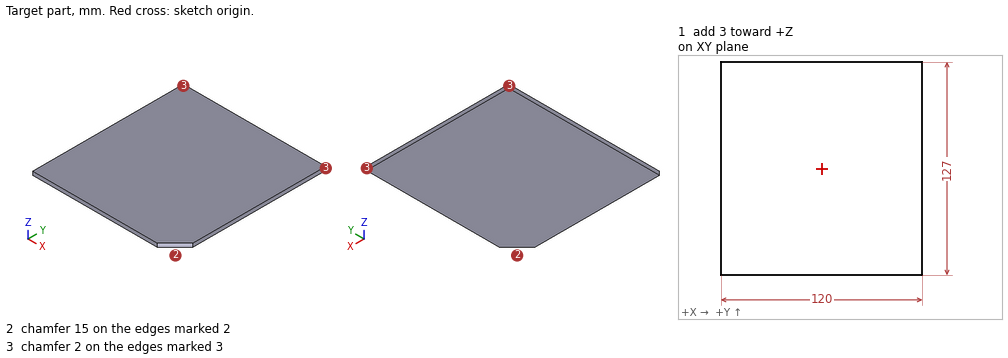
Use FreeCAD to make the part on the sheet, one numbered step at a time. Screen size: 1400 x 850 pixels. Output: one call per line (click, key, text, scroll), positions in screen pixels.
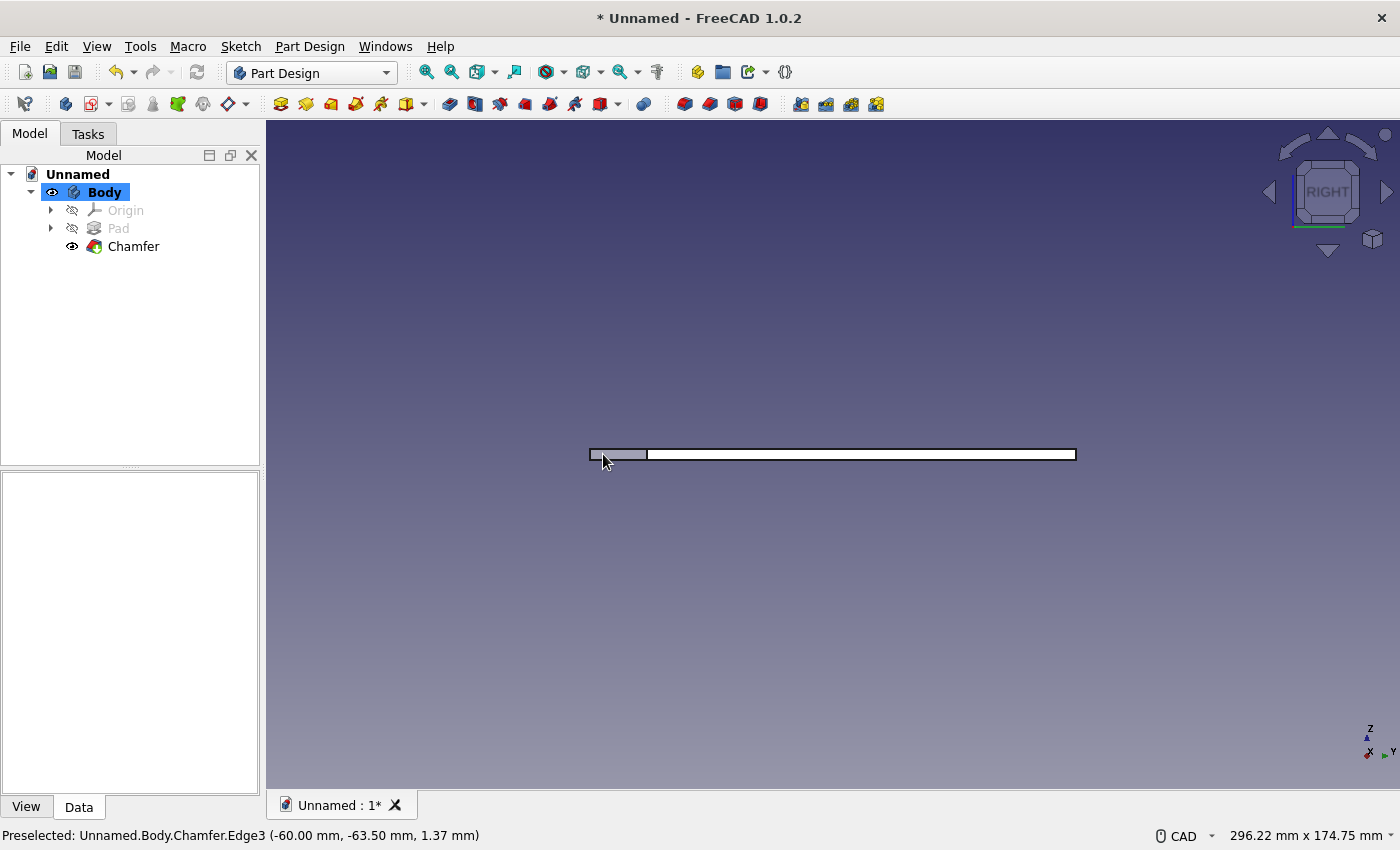
click(427, 72)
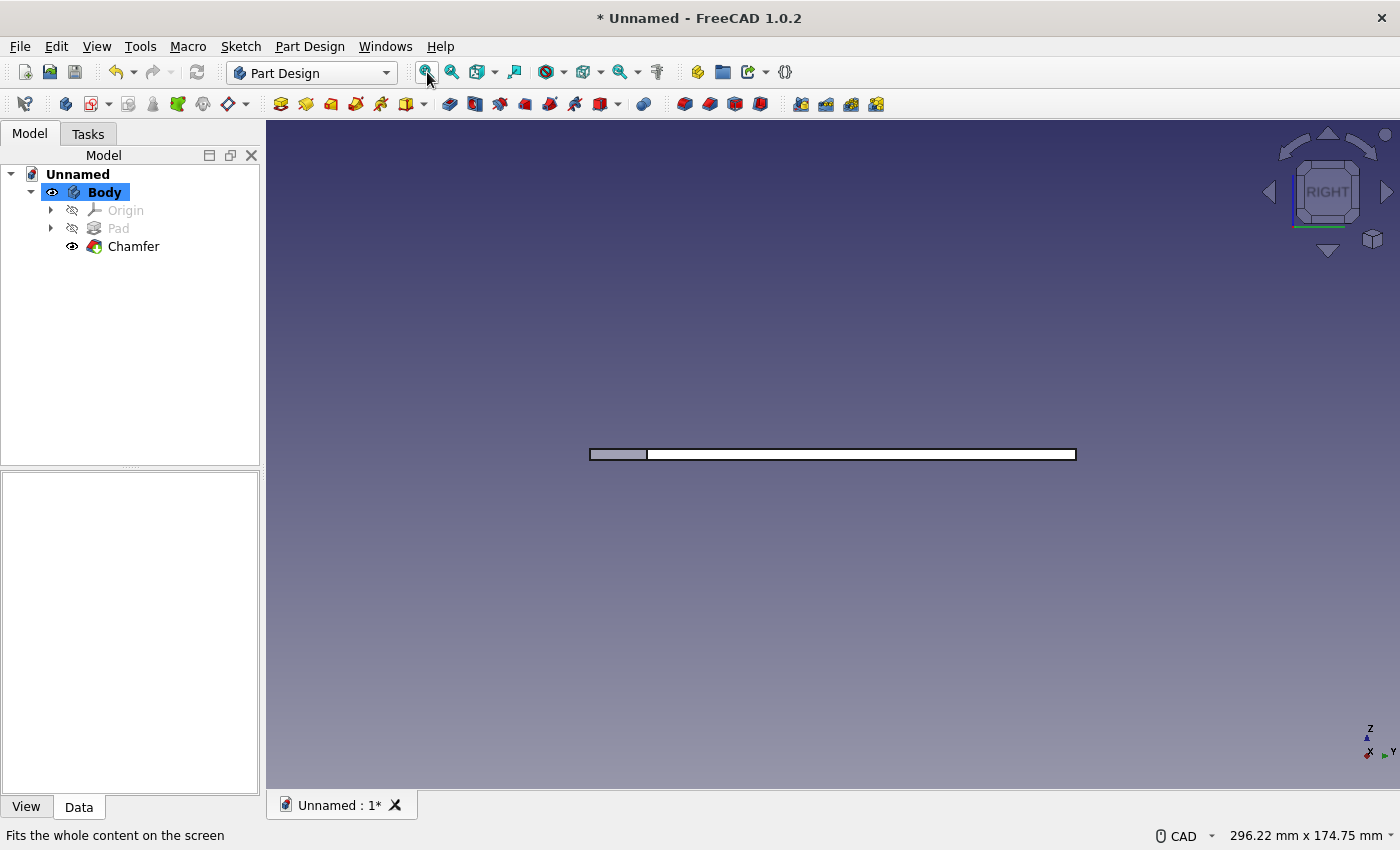
scroll(1076, 453, up, 7)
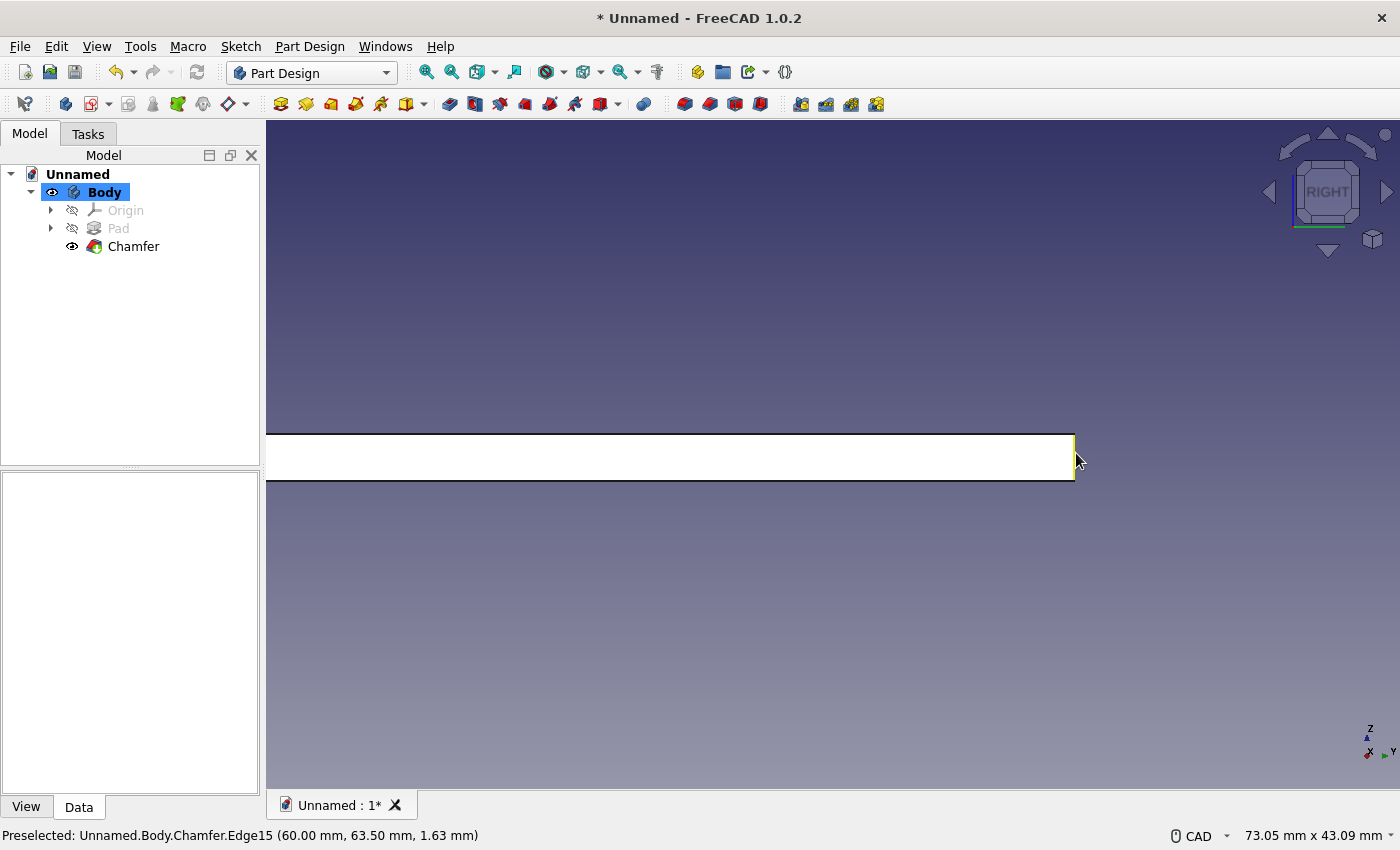
click(1074, 457)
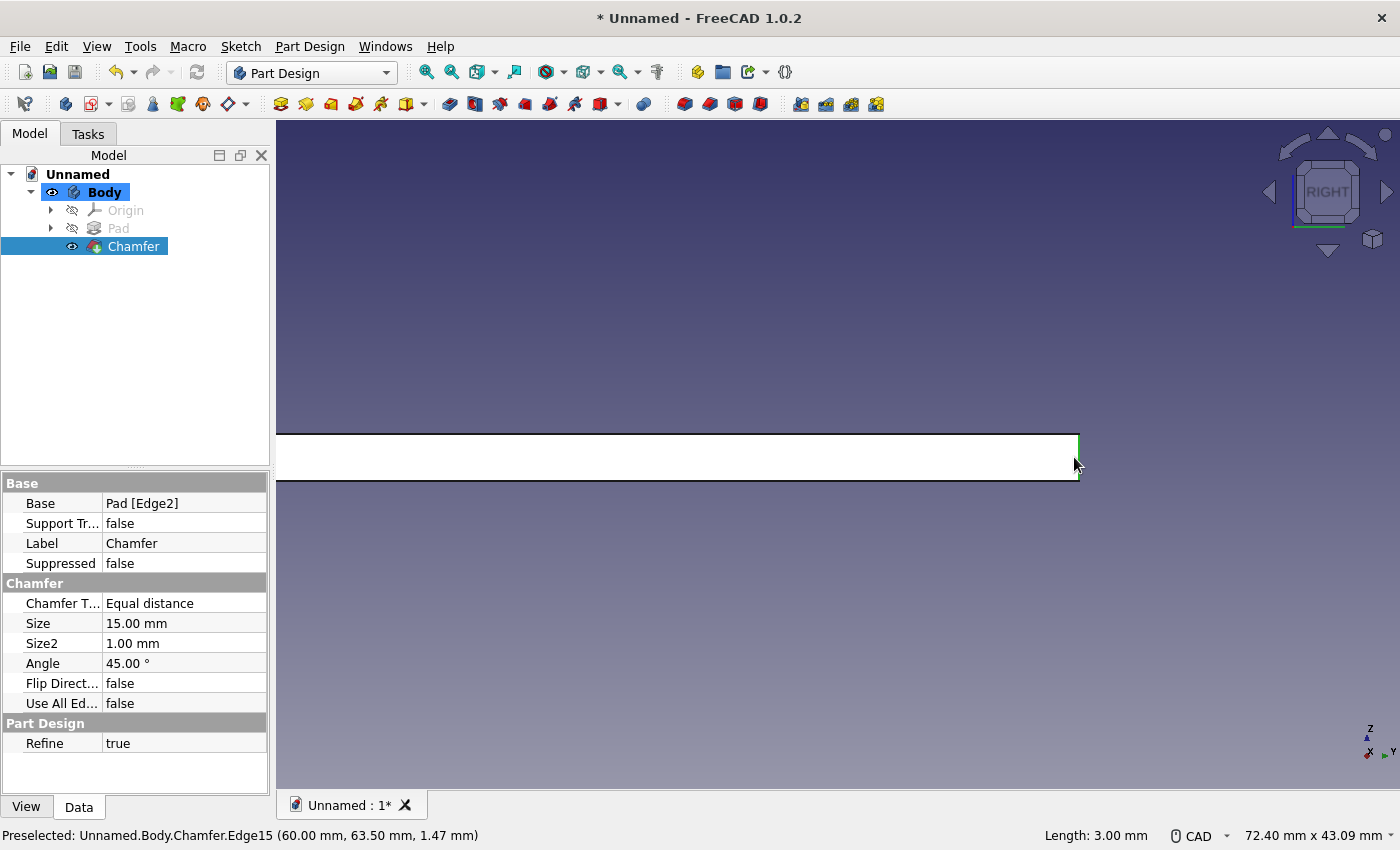
key(v)
key(f)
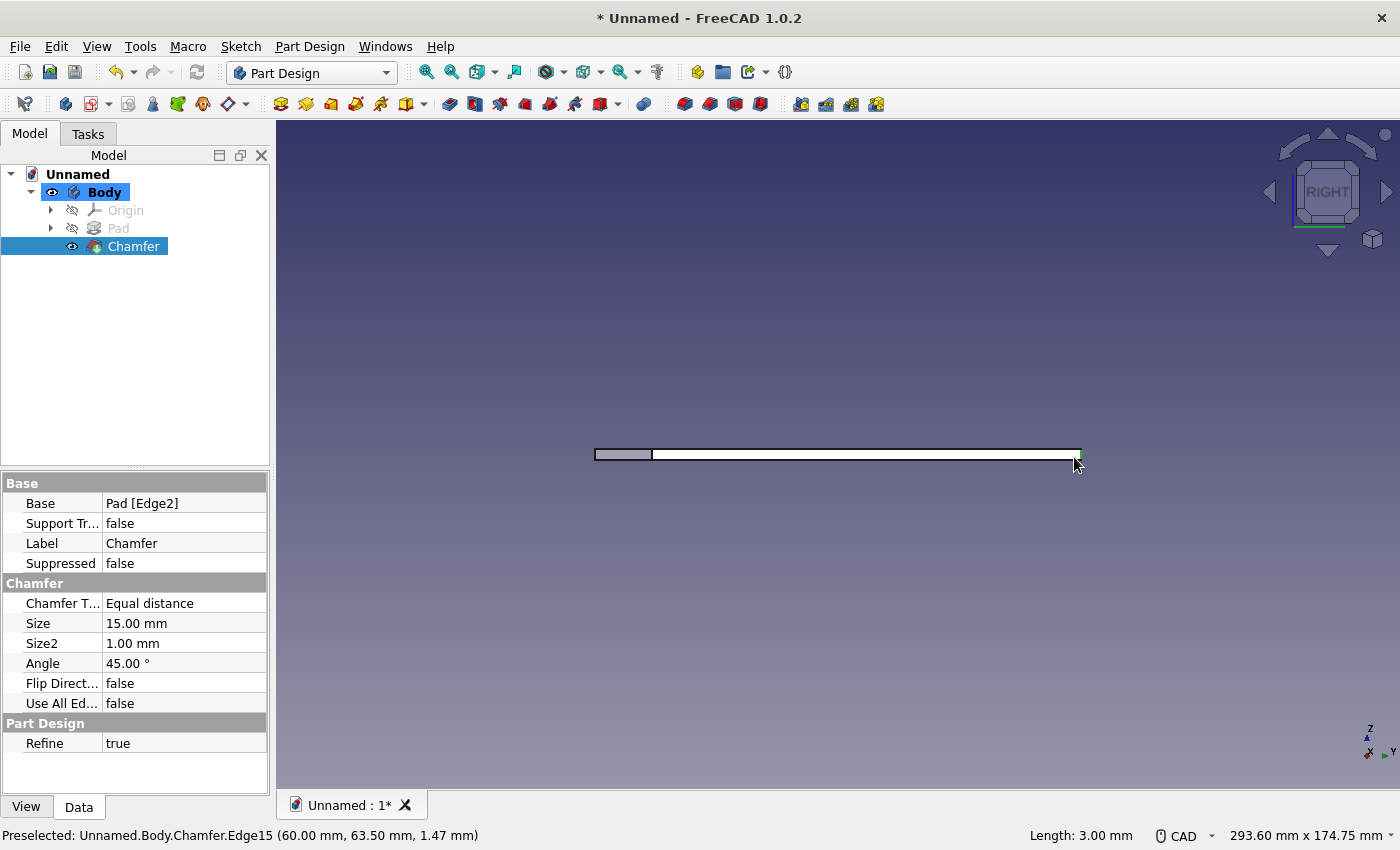
key(5)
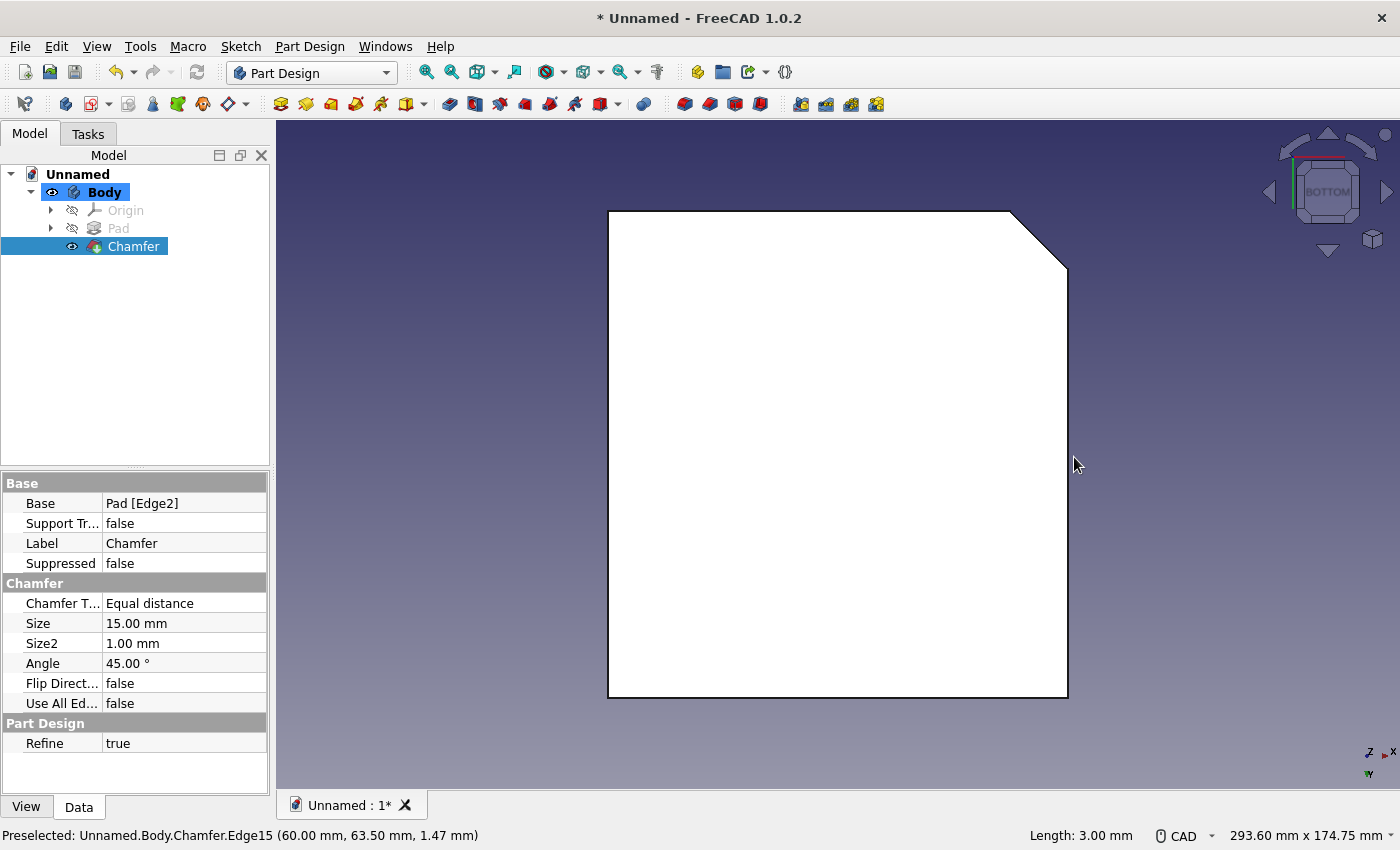
scroll(608, 697, up, 7)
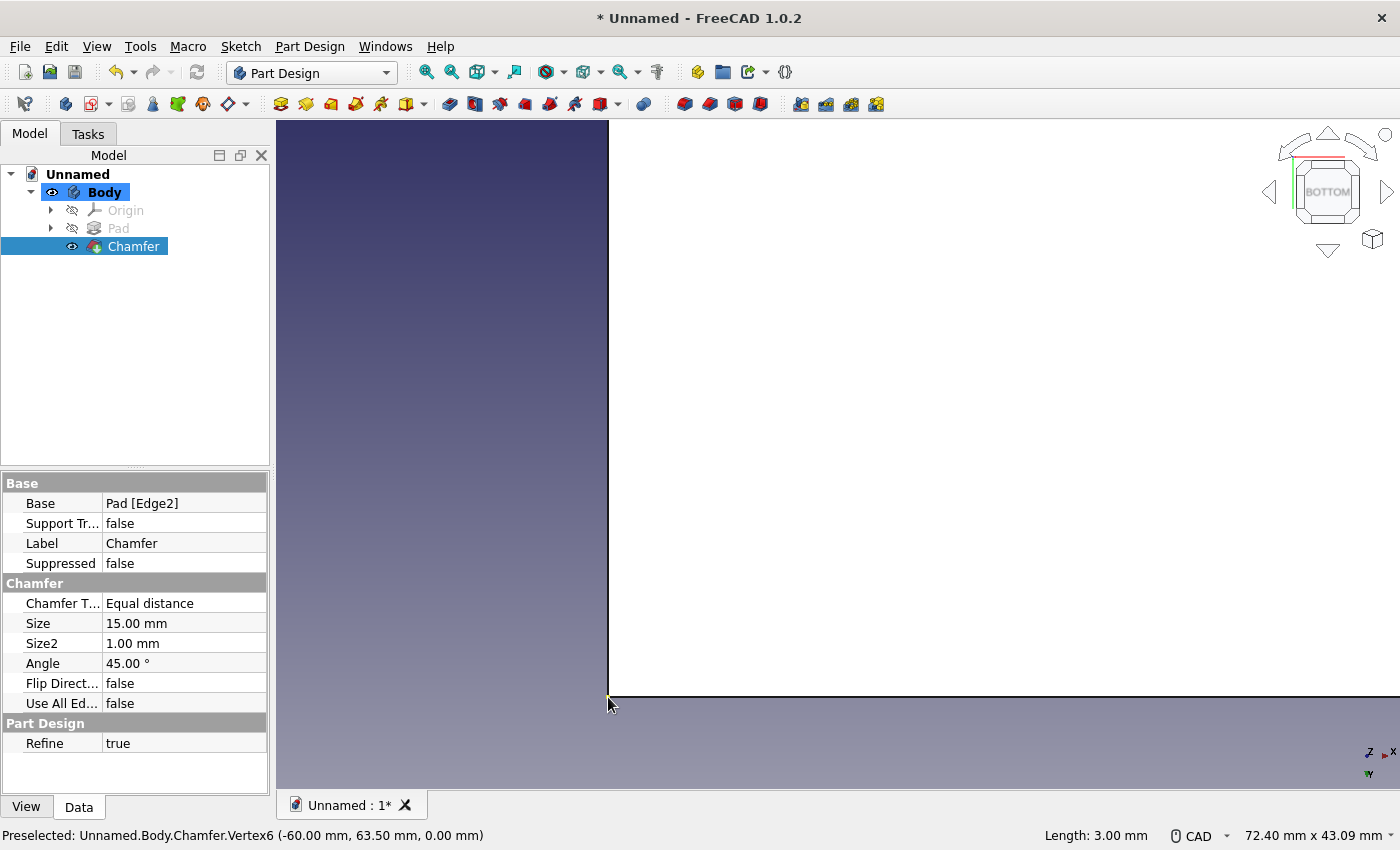
key(v)
key(f)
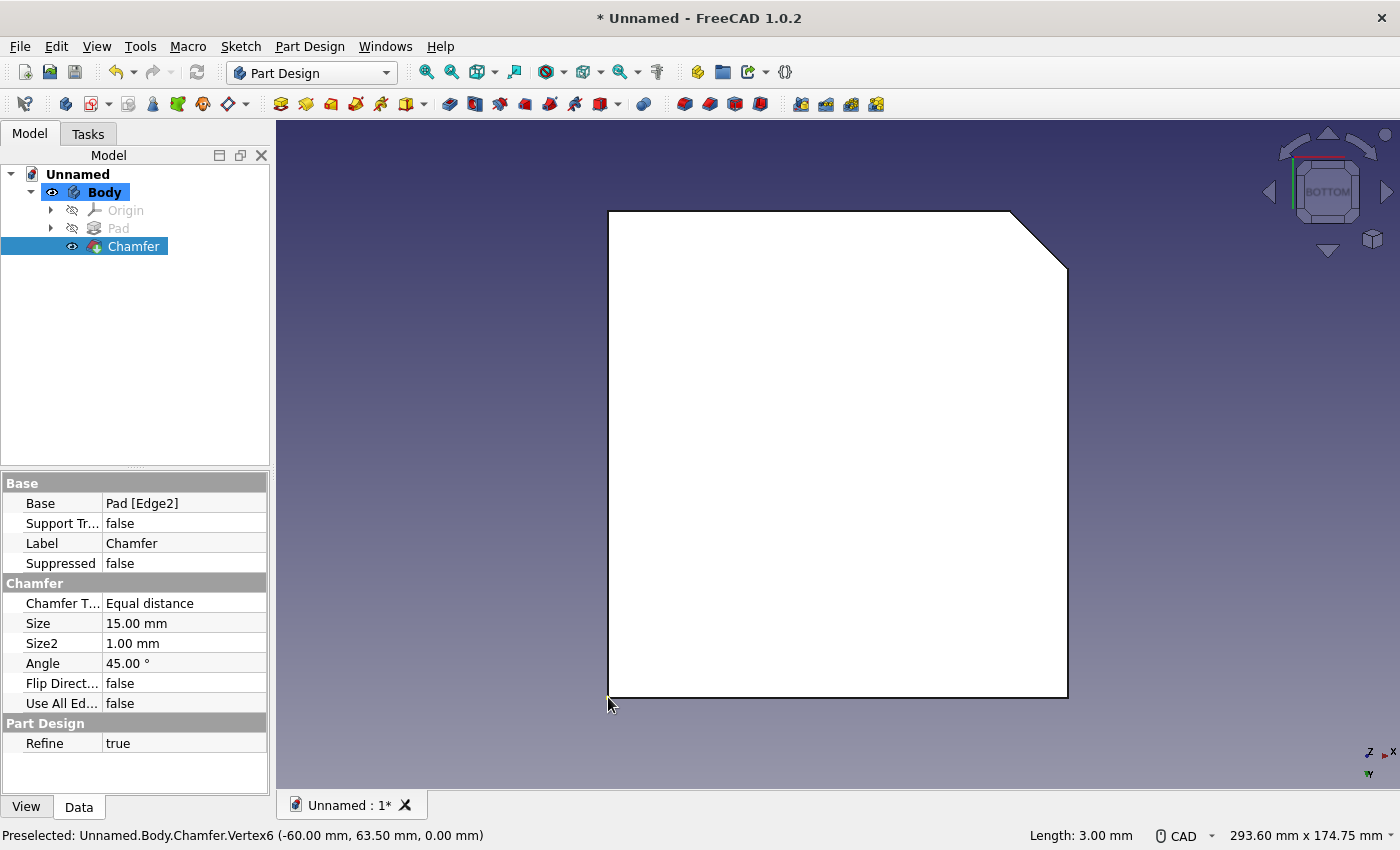
key(4)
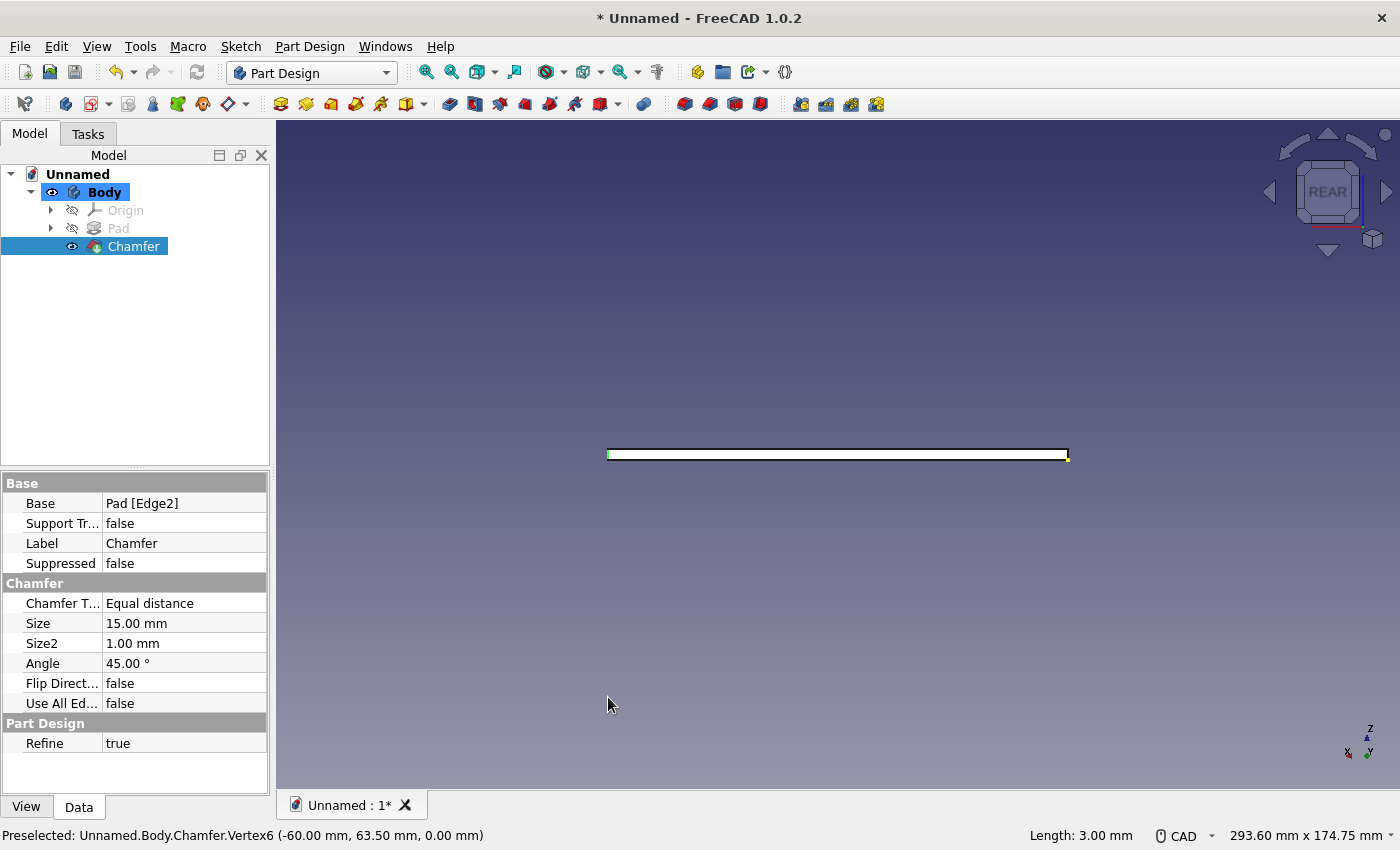
key(v)
key(f)